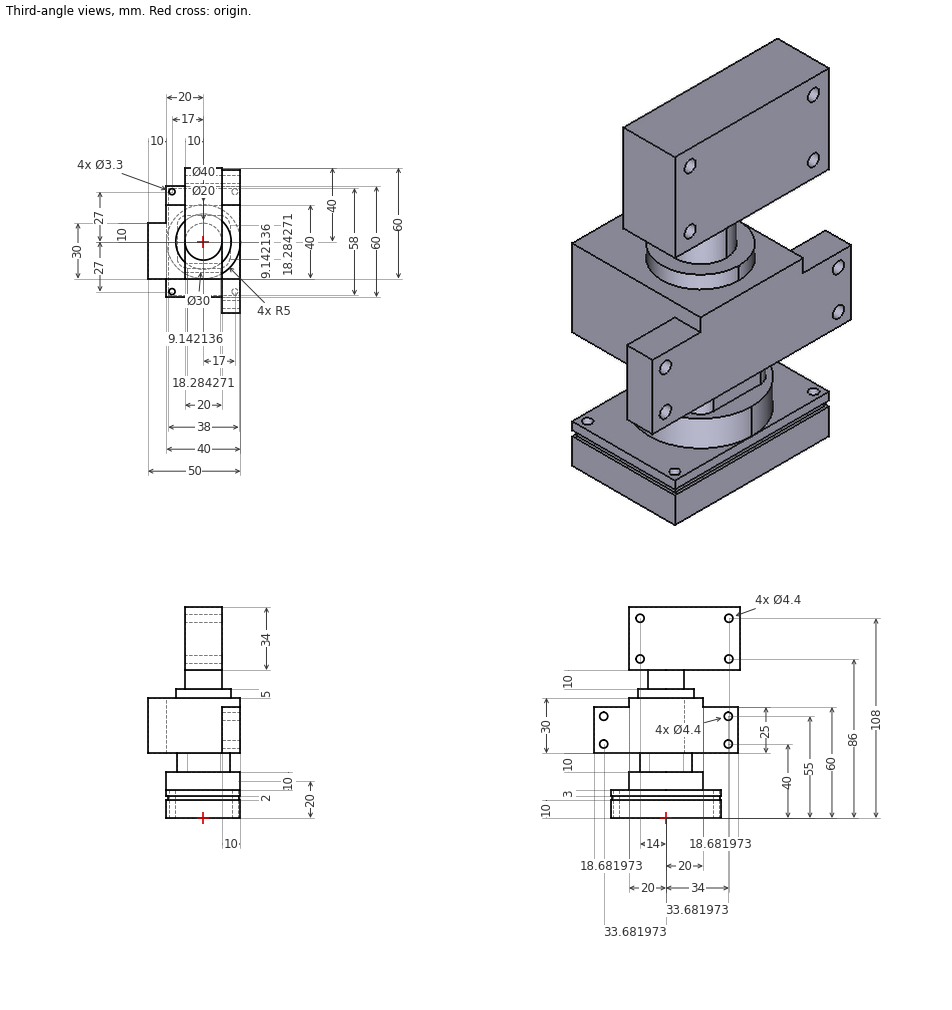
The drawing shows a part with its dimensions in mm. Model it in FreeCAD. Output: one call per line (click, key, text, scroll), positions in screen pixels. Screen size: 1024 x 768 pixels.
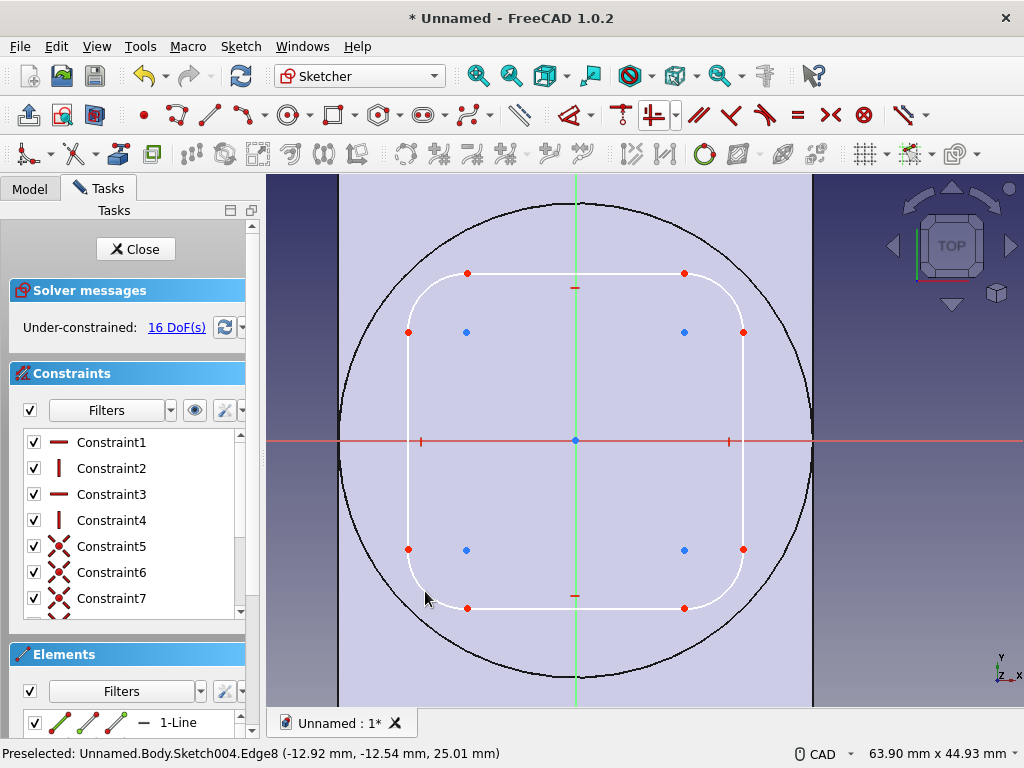
click(532, 609)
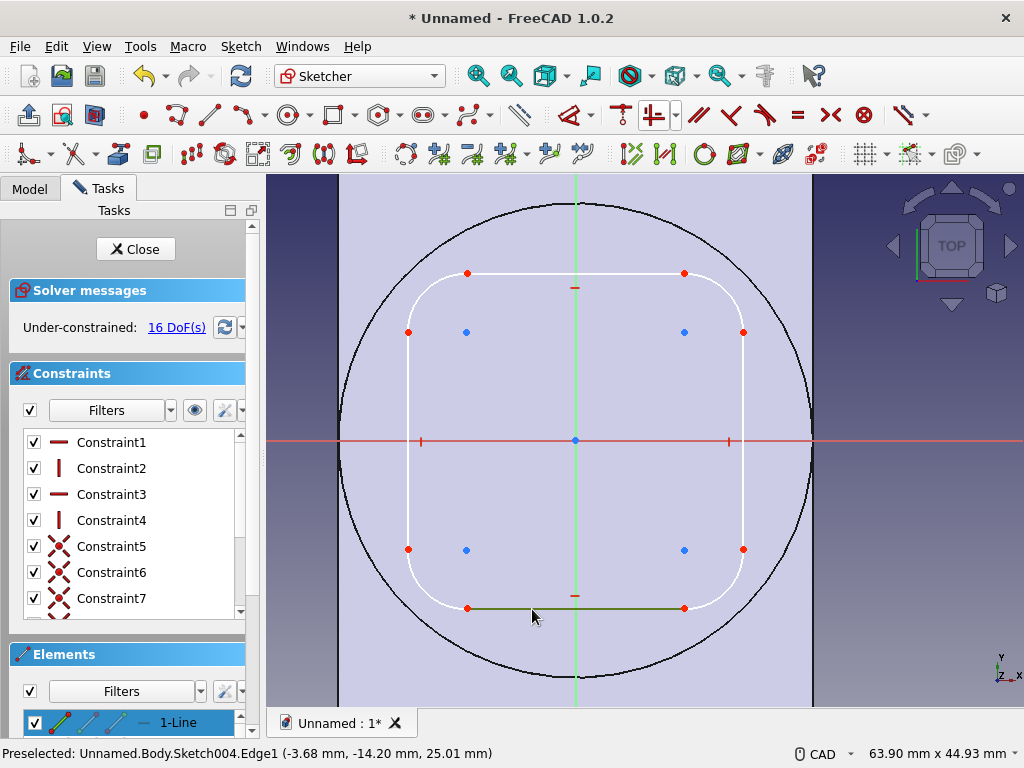
click(711, 603)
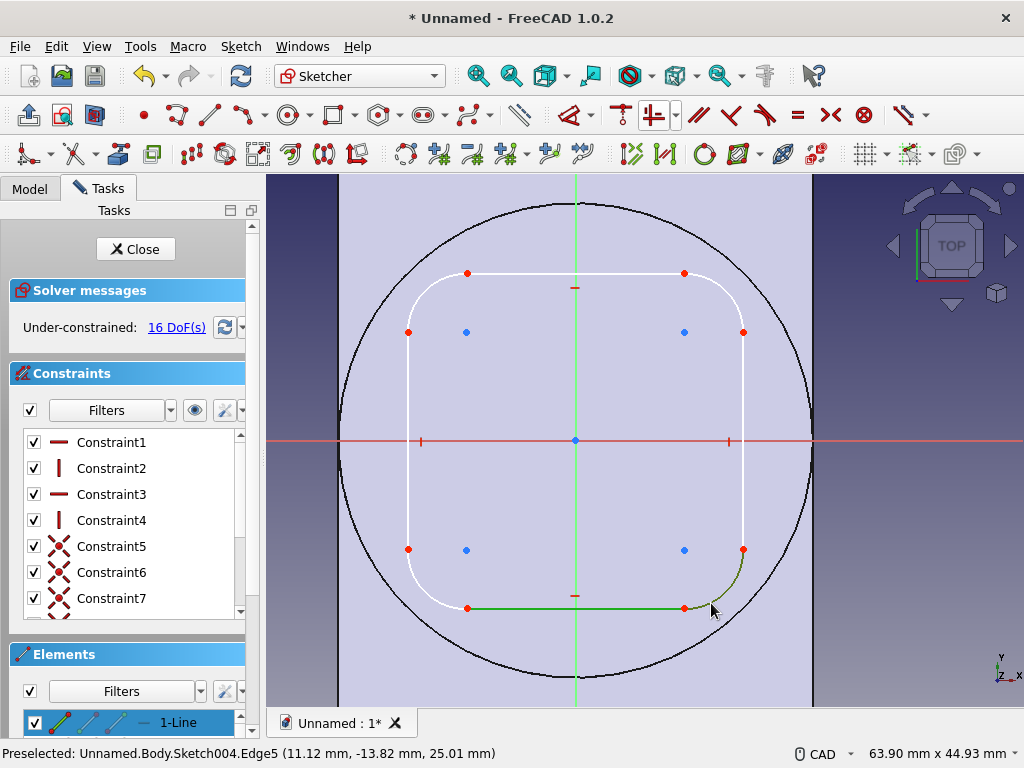
click(765, 116)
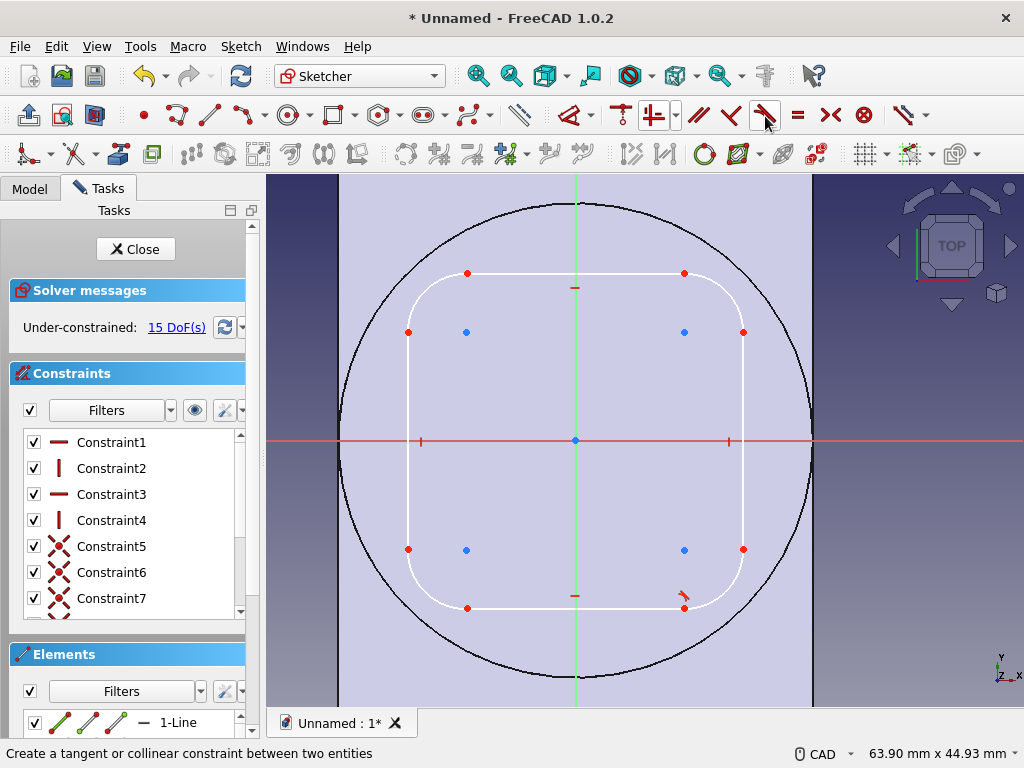
click(532, 609)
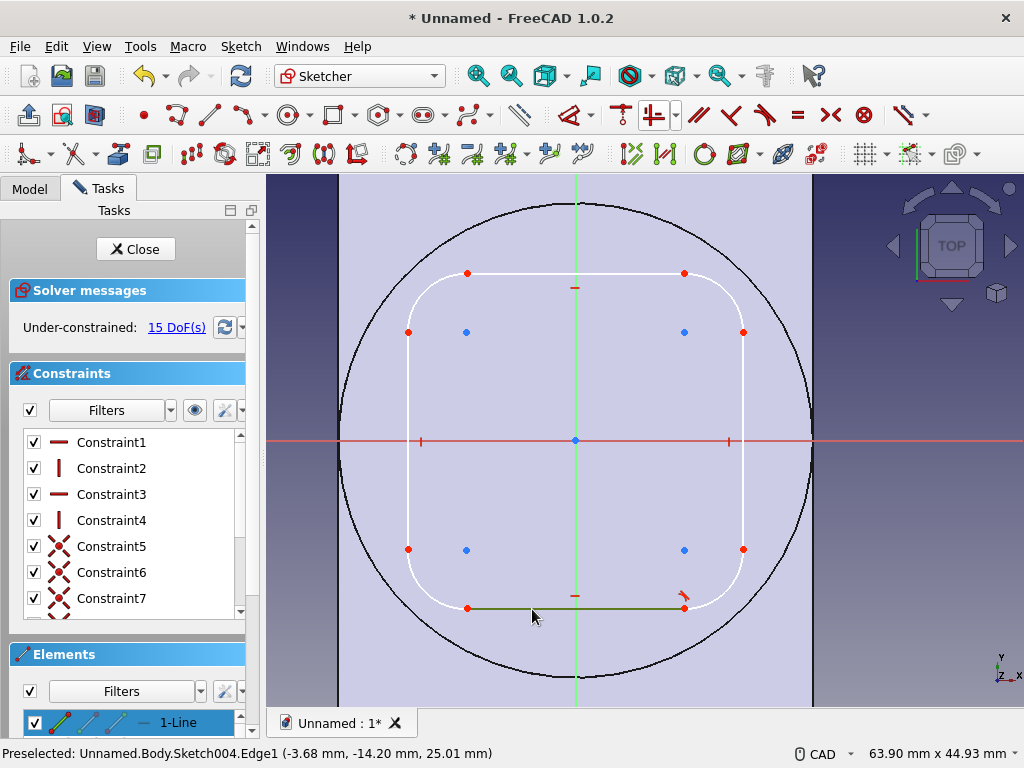
click(414, 577)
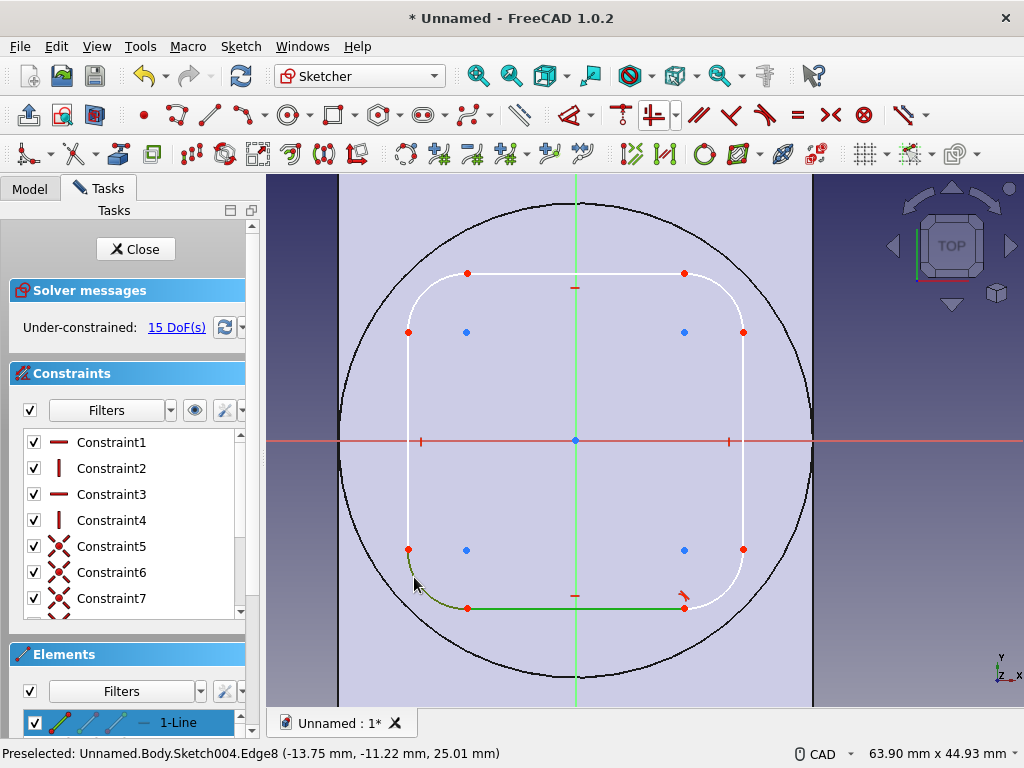
click(765, 116)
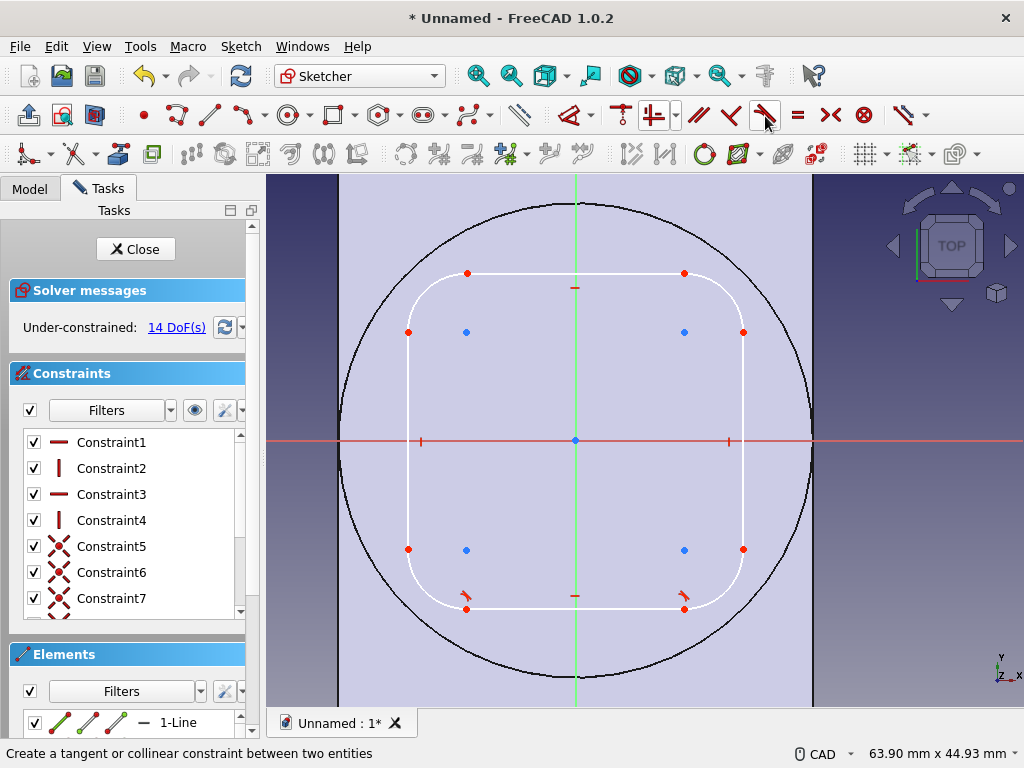
click(743, 485)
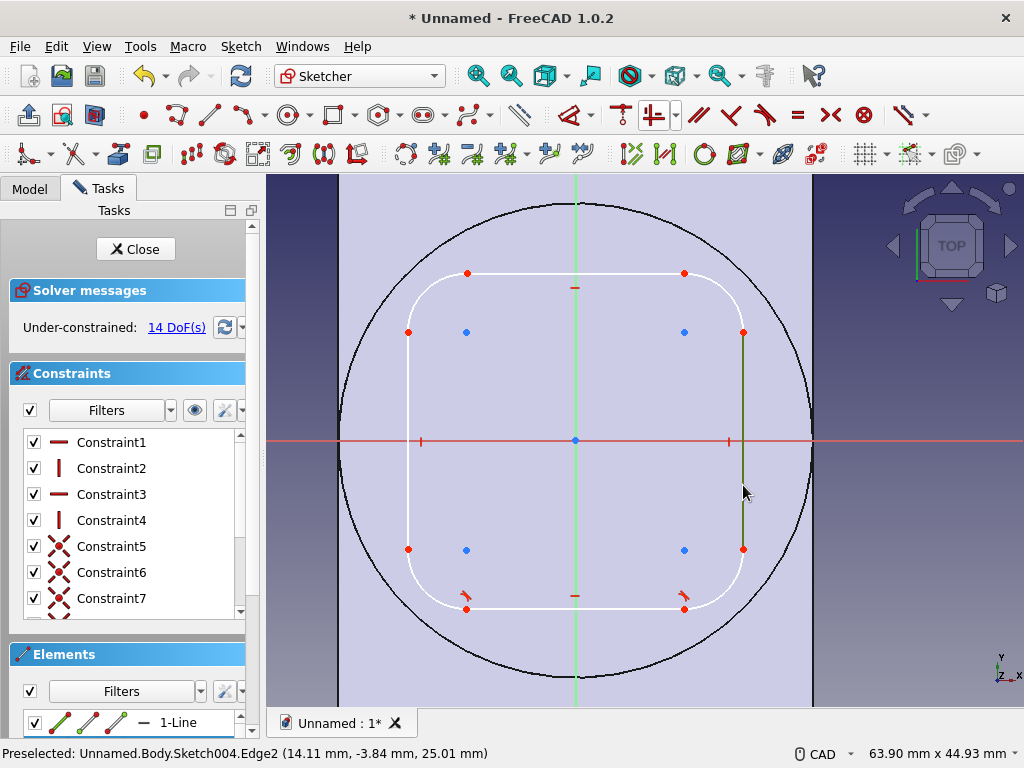
click(711, 603)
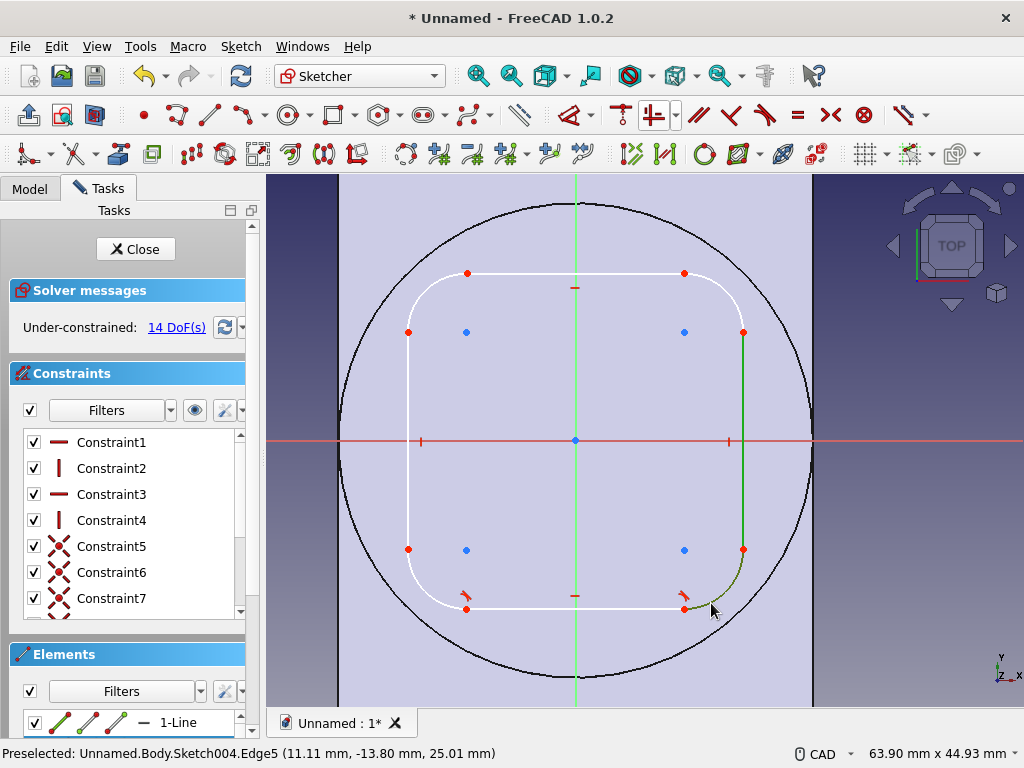
key(t)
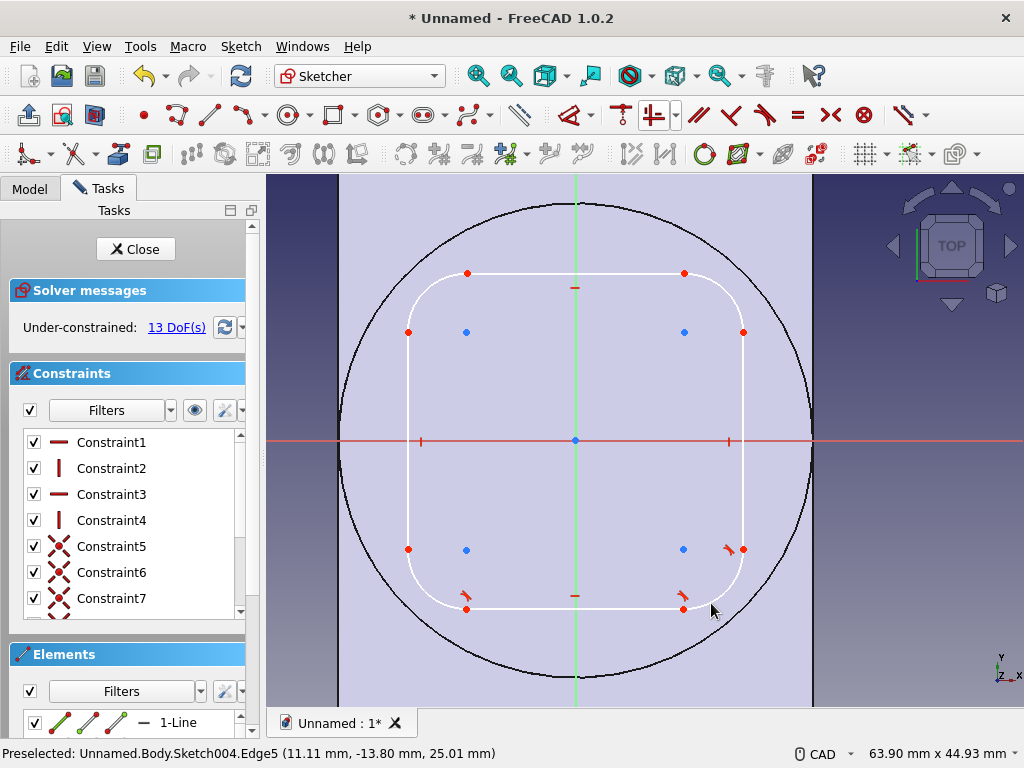
click(743, 485)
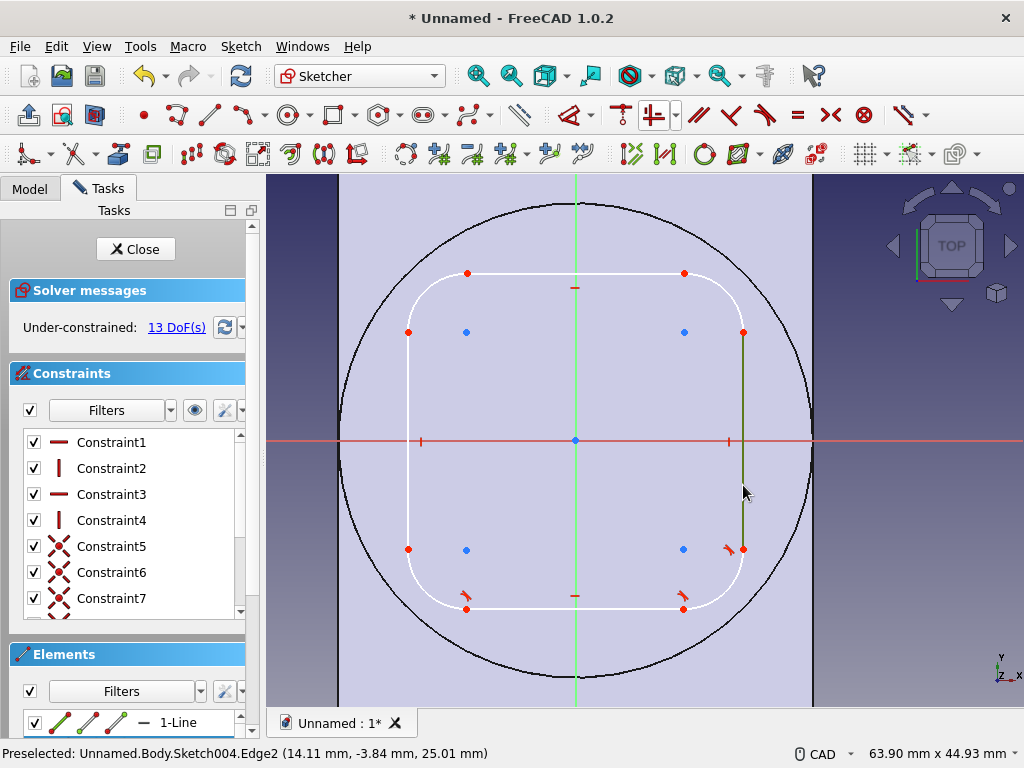
click(737, 306)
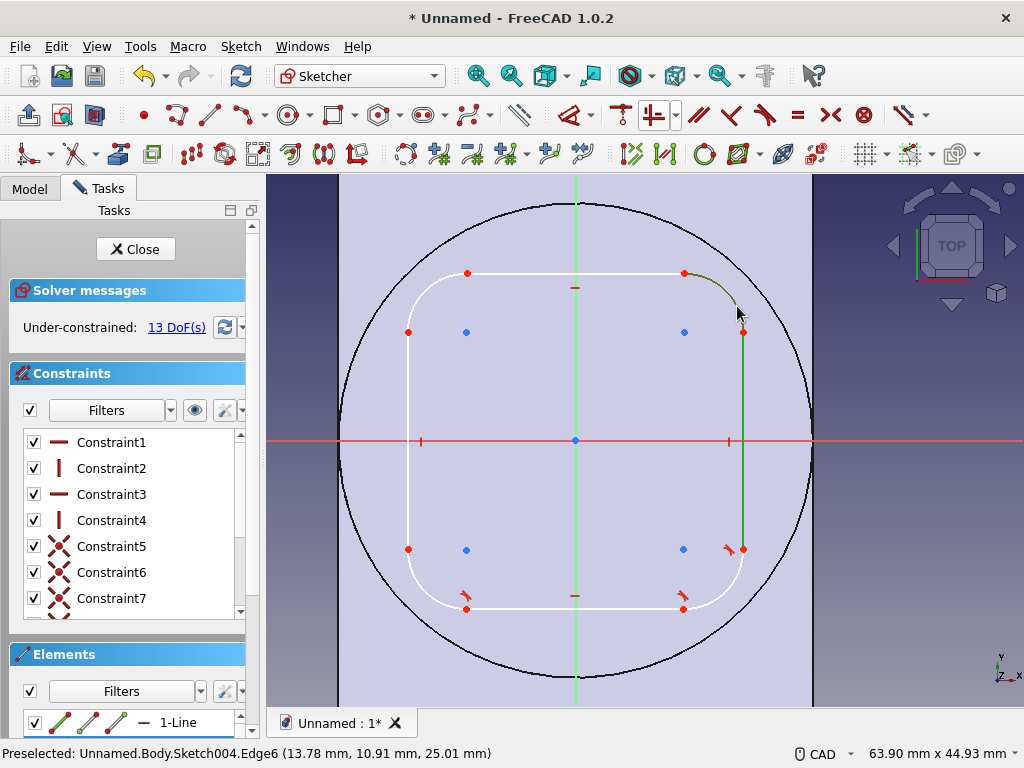
key(t)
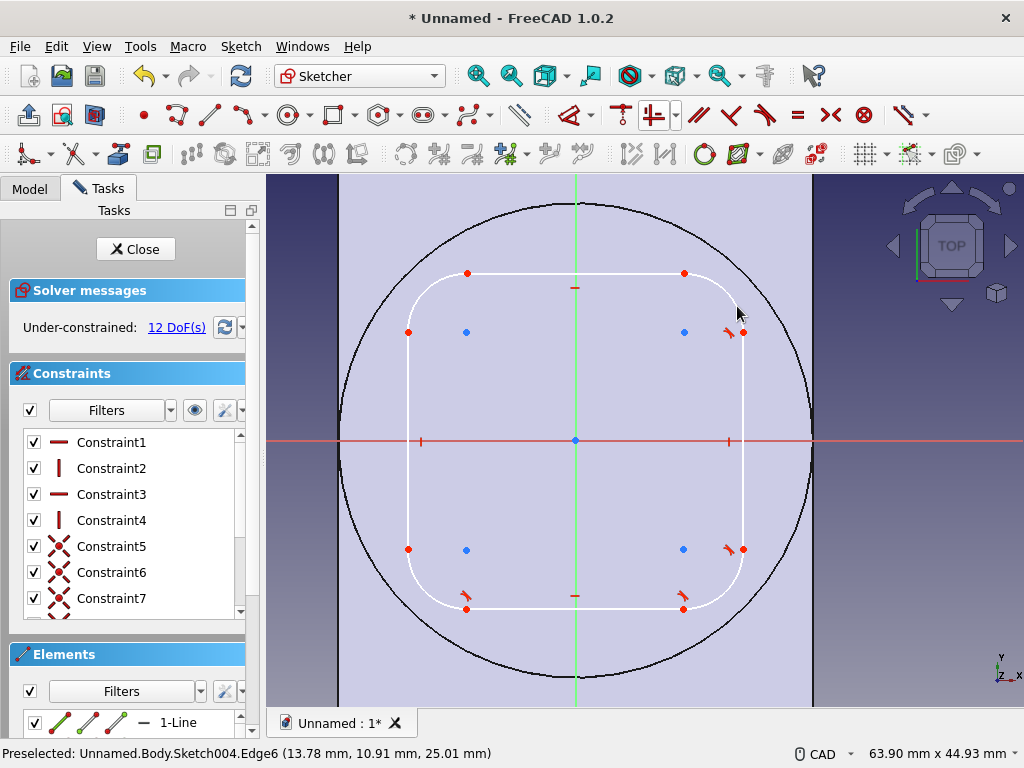
click(619, 274)